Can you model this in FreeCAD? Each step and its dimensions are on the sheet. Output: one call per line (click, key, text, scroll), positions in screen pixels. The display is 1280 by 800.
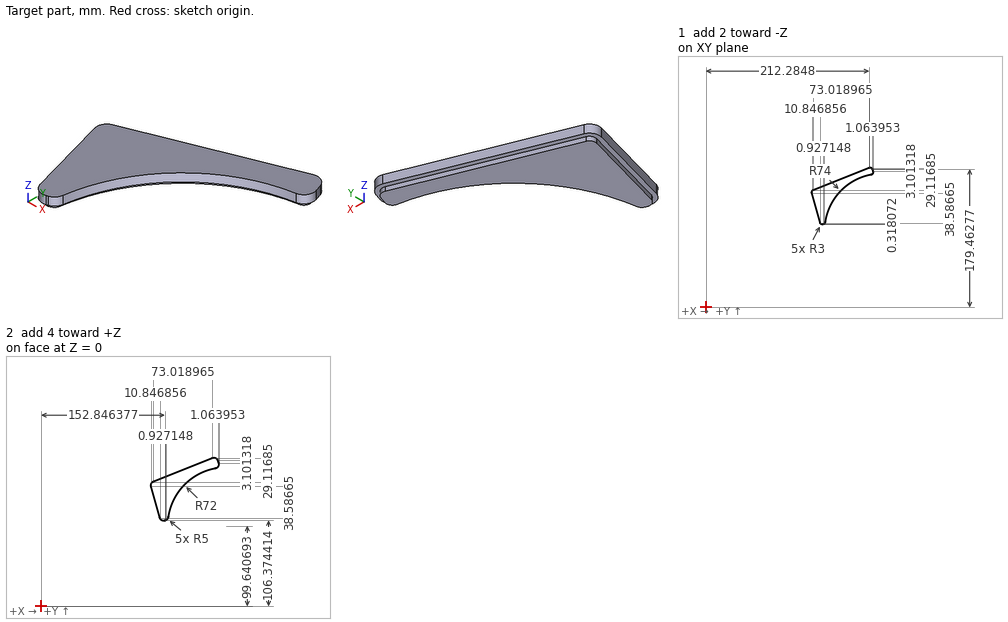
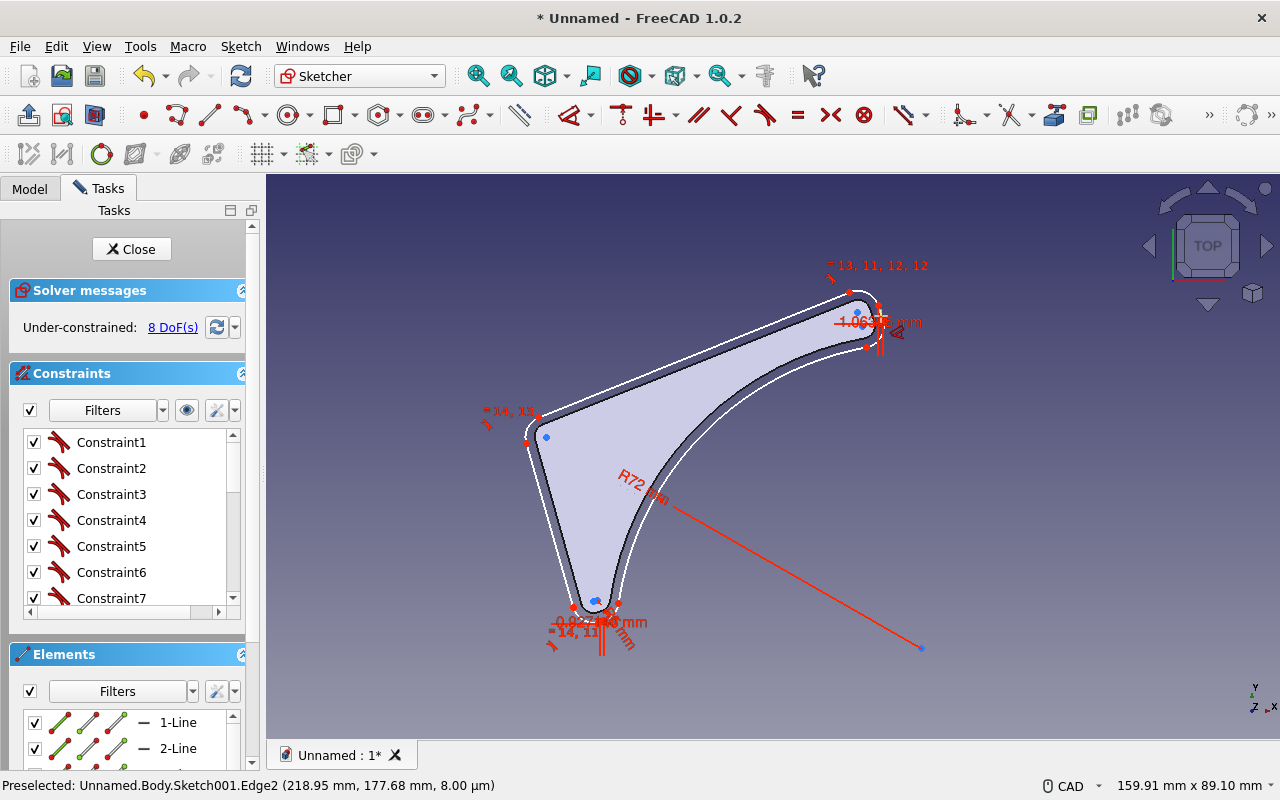
scroll(881, 316, up, 6)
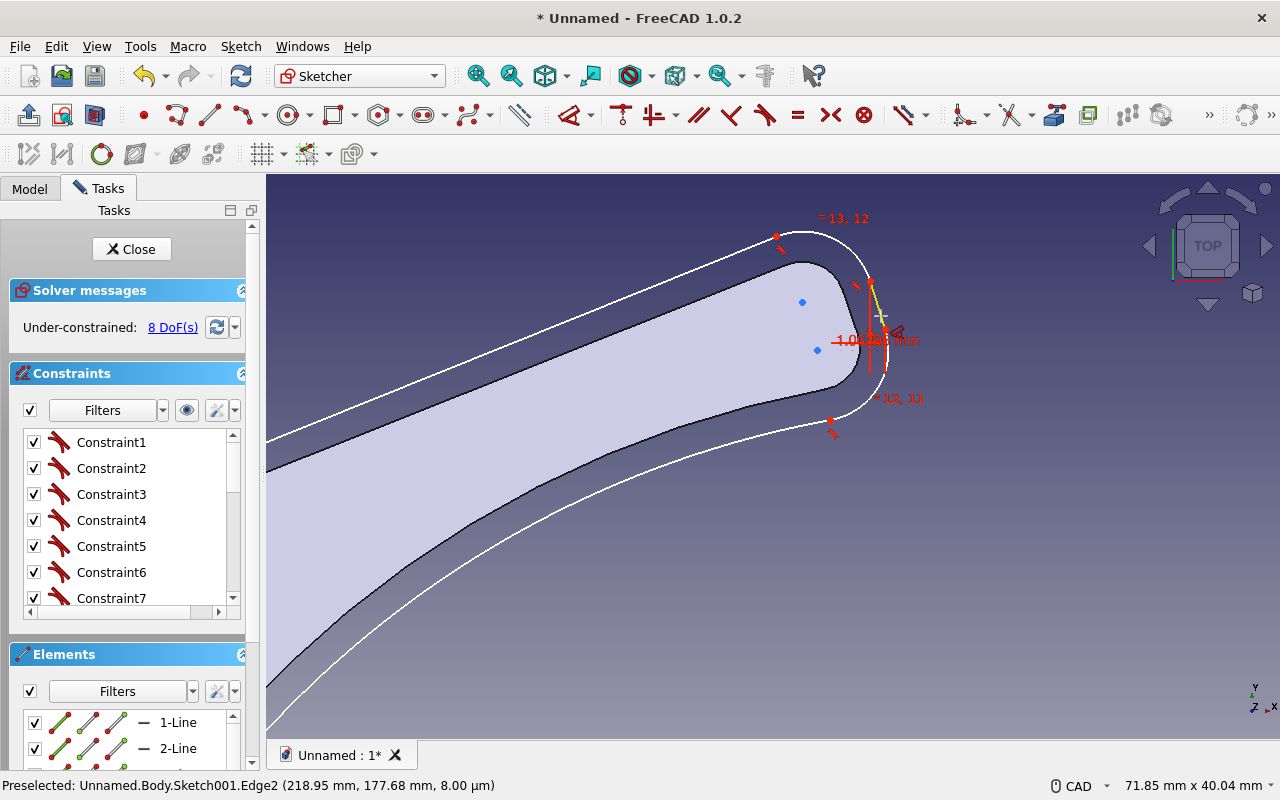
click(881, 315)
click(919, 305)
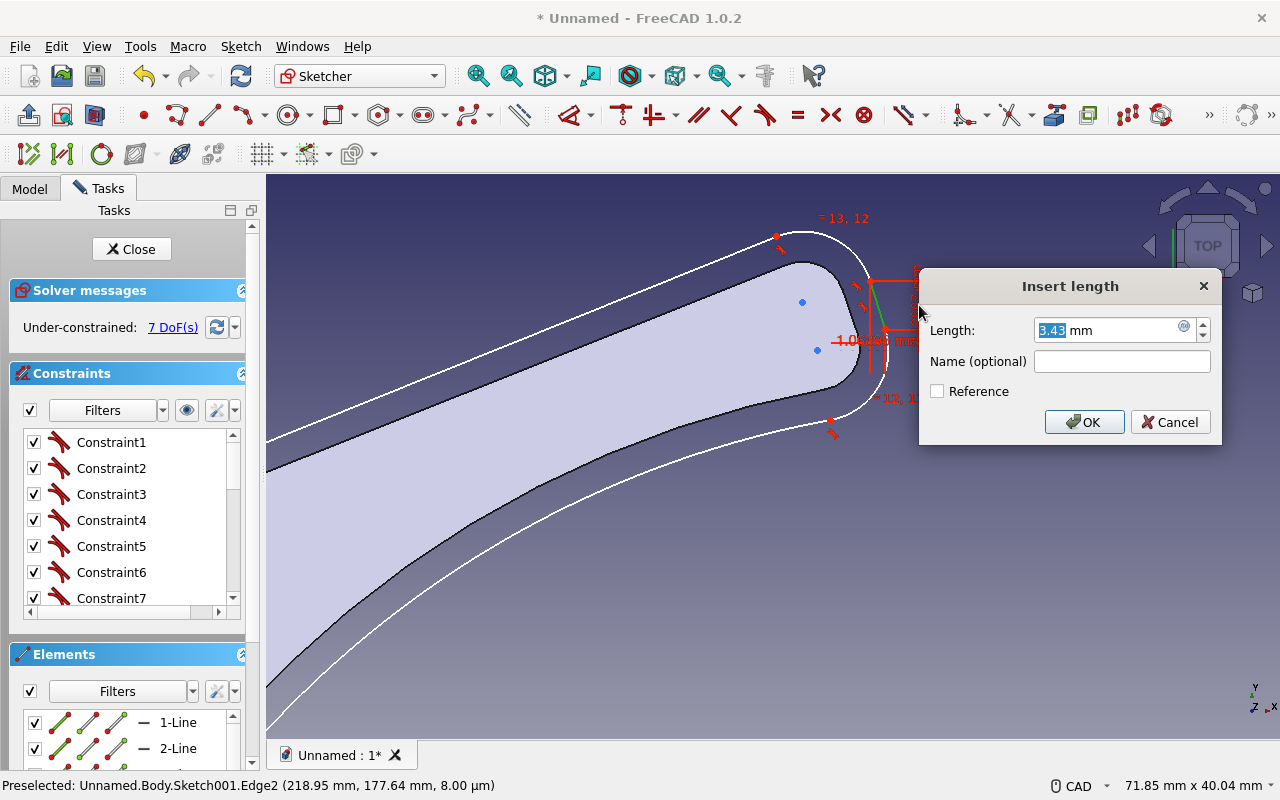
text(3.101318)
key(Return)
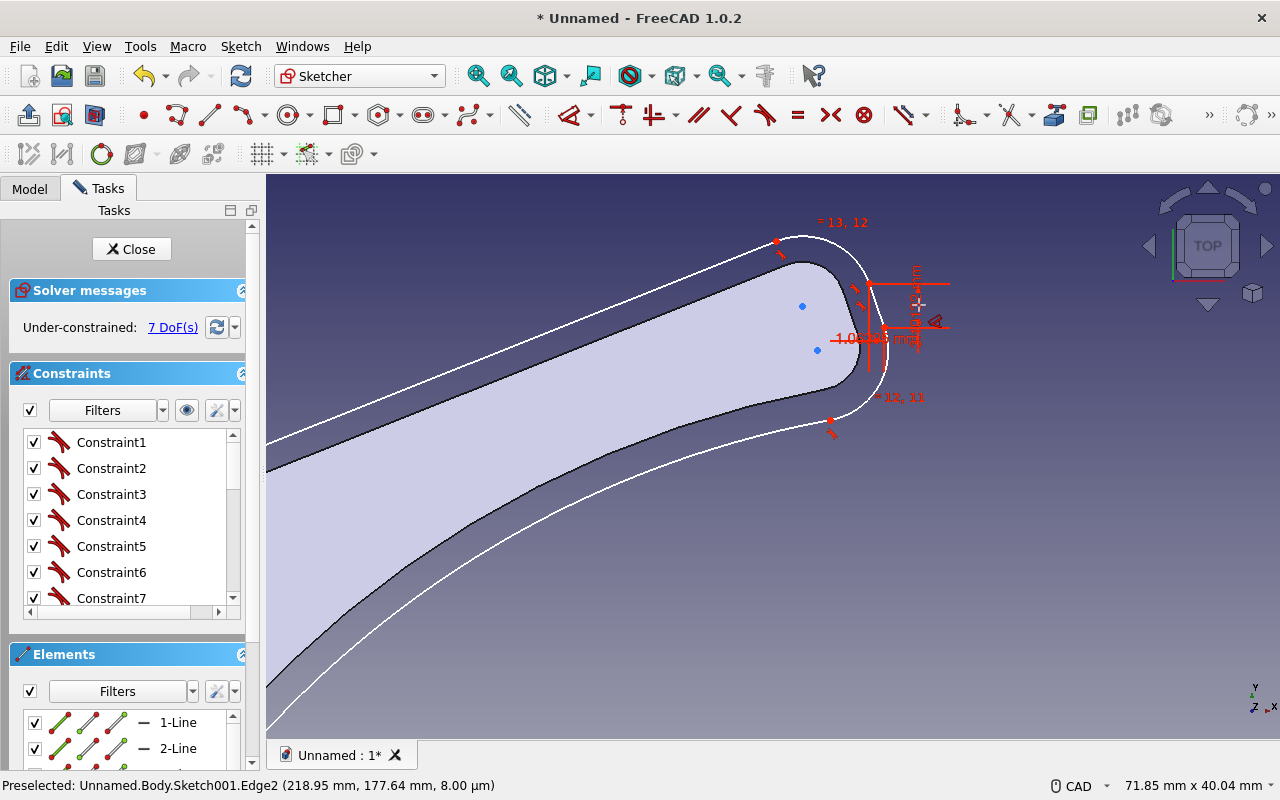
click(467, 365)
click(810, 447)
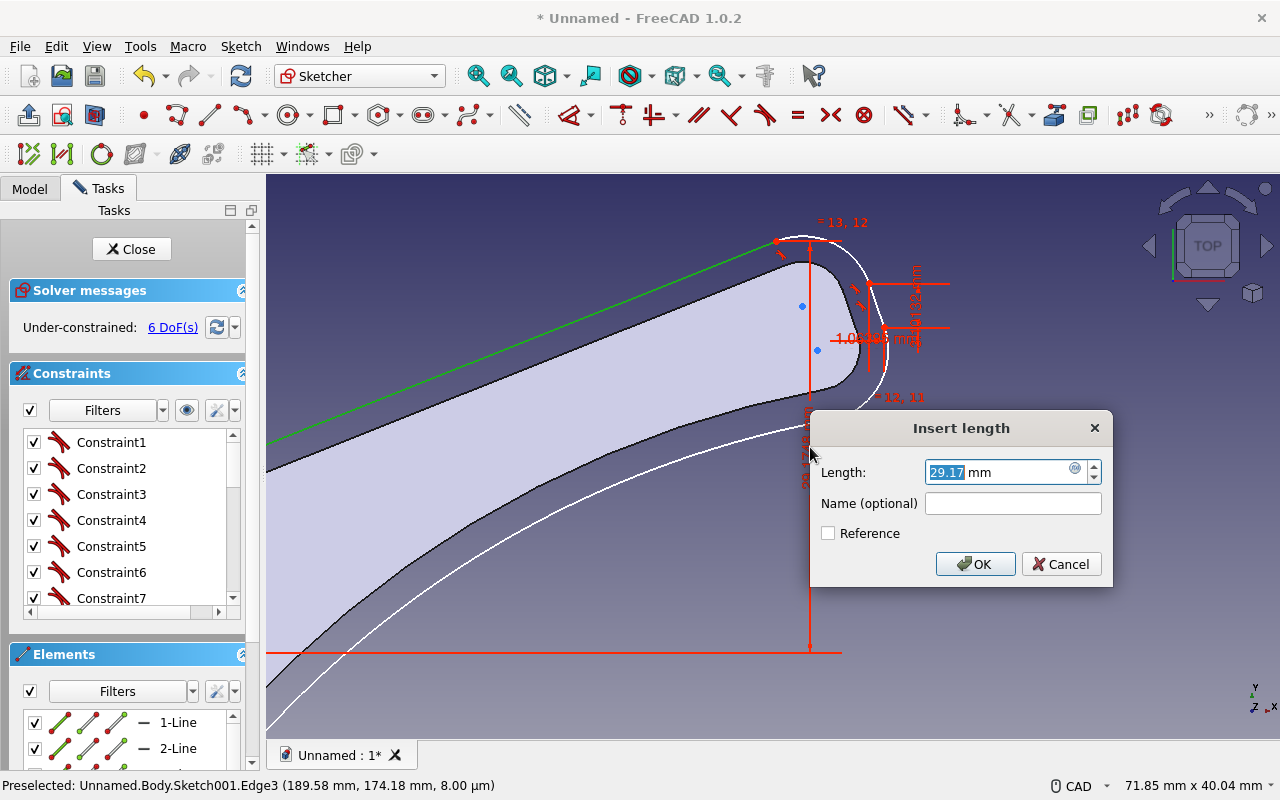
text(29.11685)
key(Return)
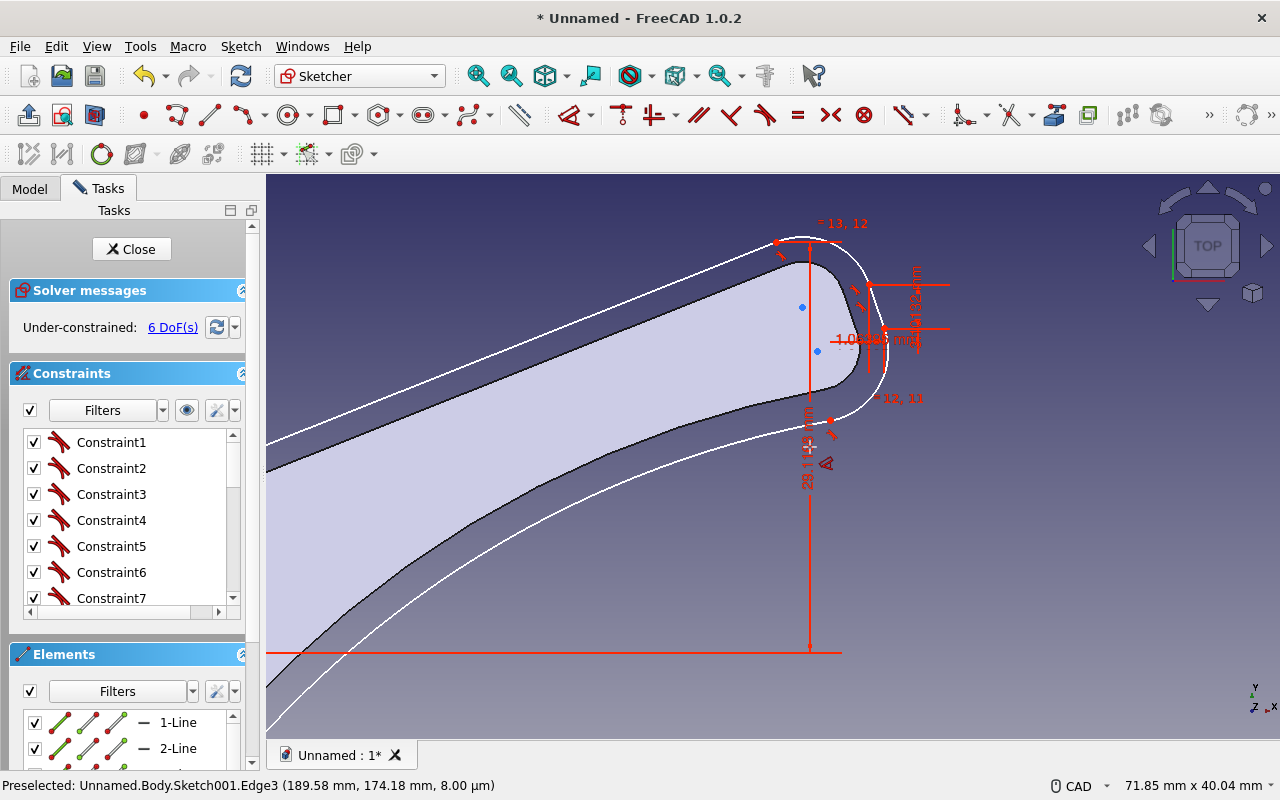
scroll(881, 316, down, 6)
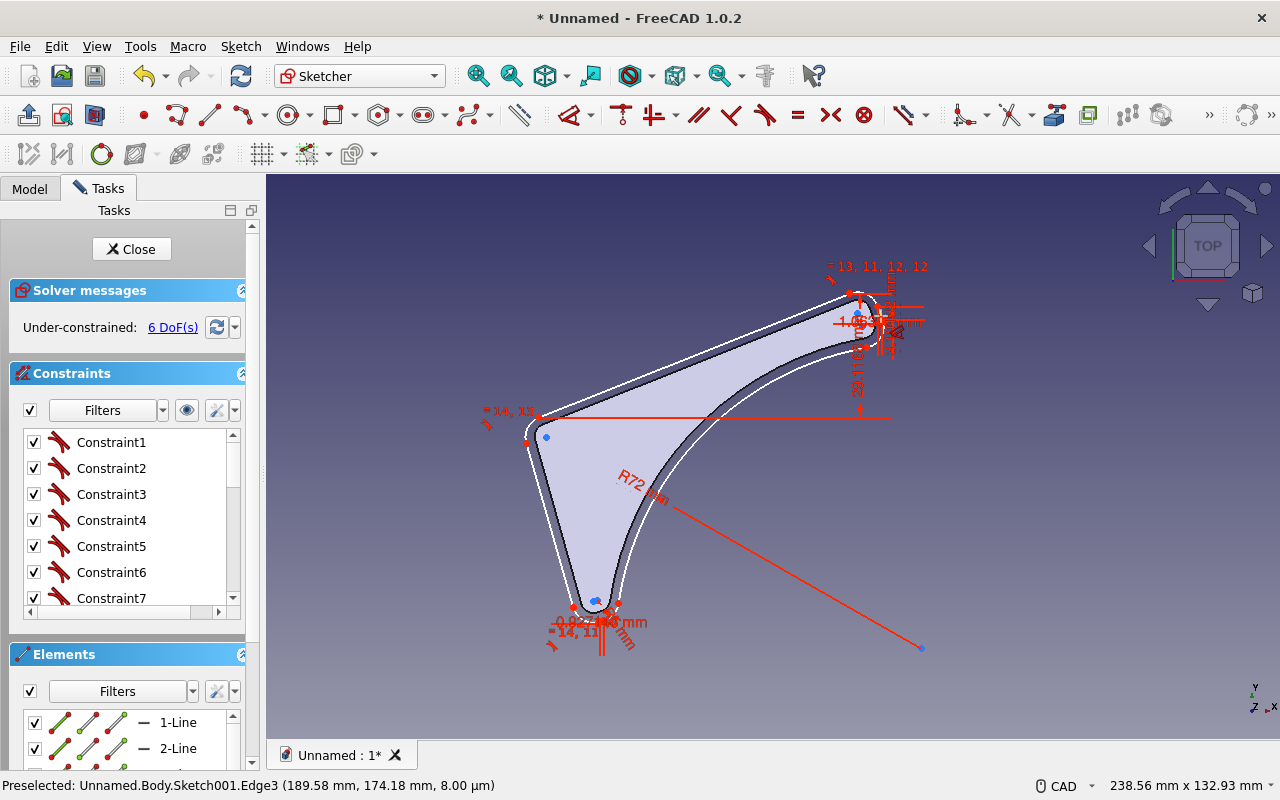
click(540, 492)
click(492, 525)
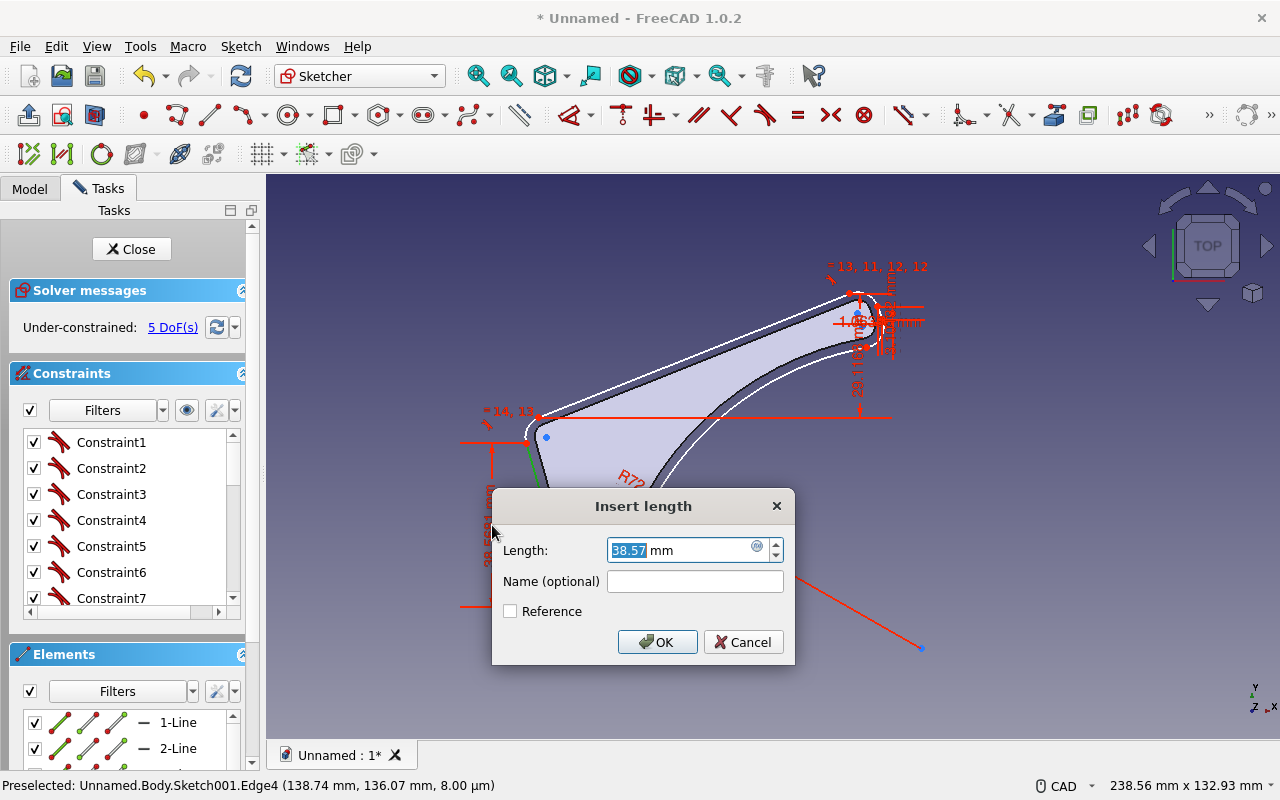
text(38.58665)
key(Return)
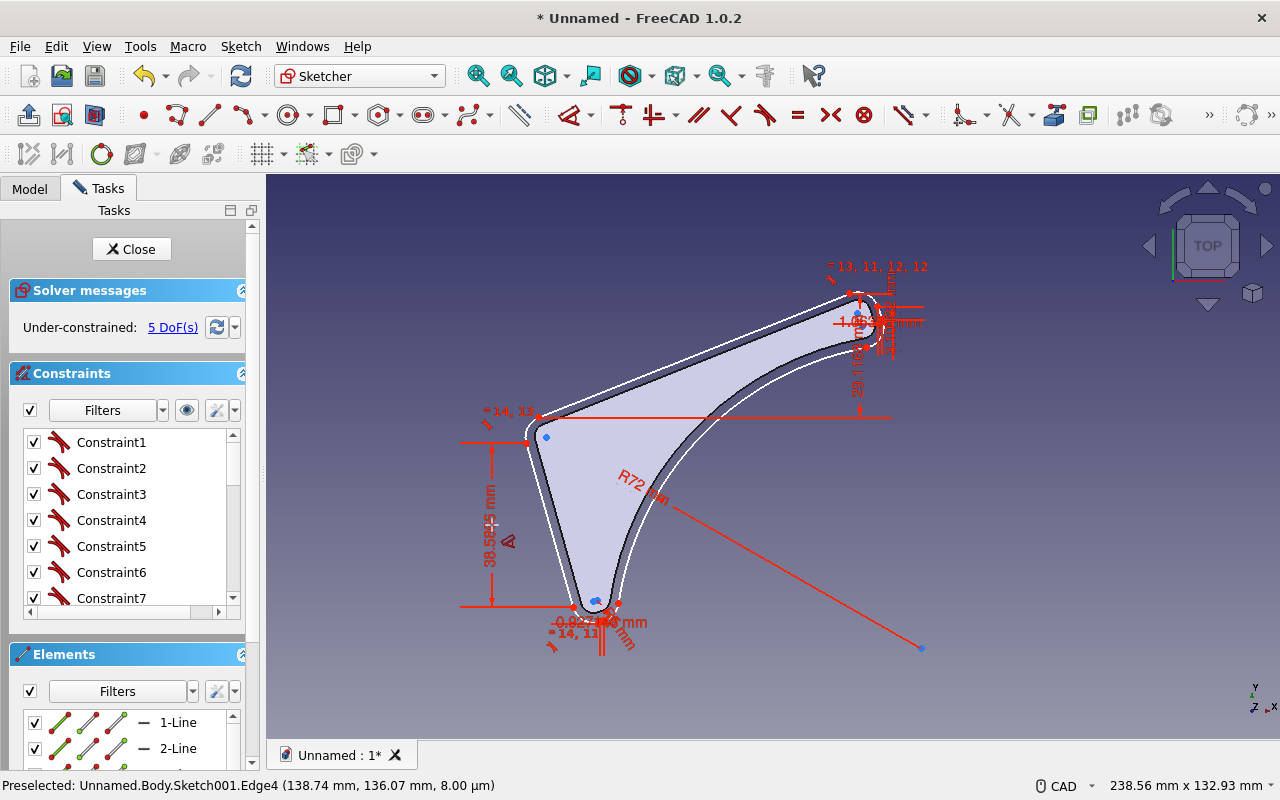
click(757, 331)
click(694, 260)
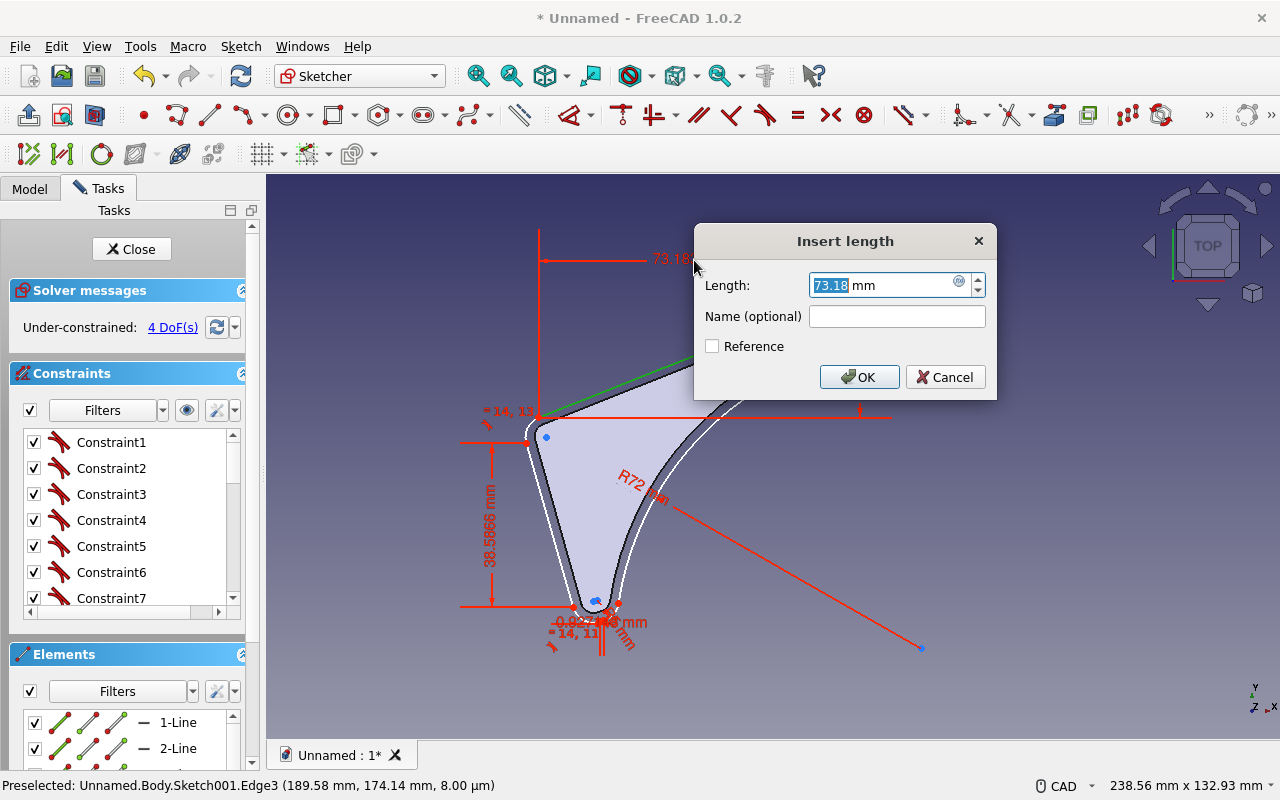
text(73.018965)
key(Return)